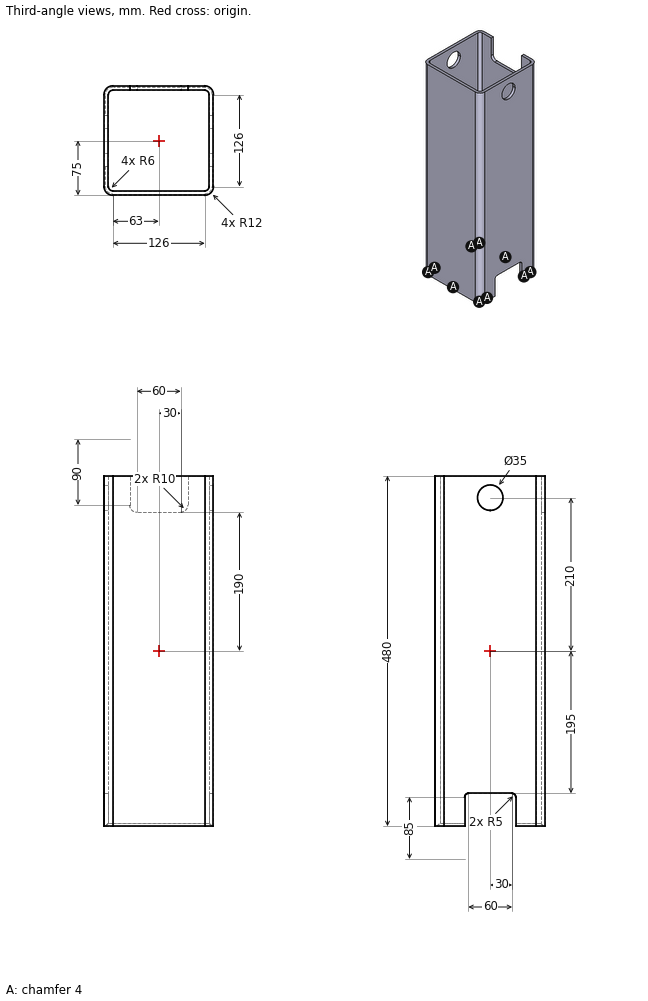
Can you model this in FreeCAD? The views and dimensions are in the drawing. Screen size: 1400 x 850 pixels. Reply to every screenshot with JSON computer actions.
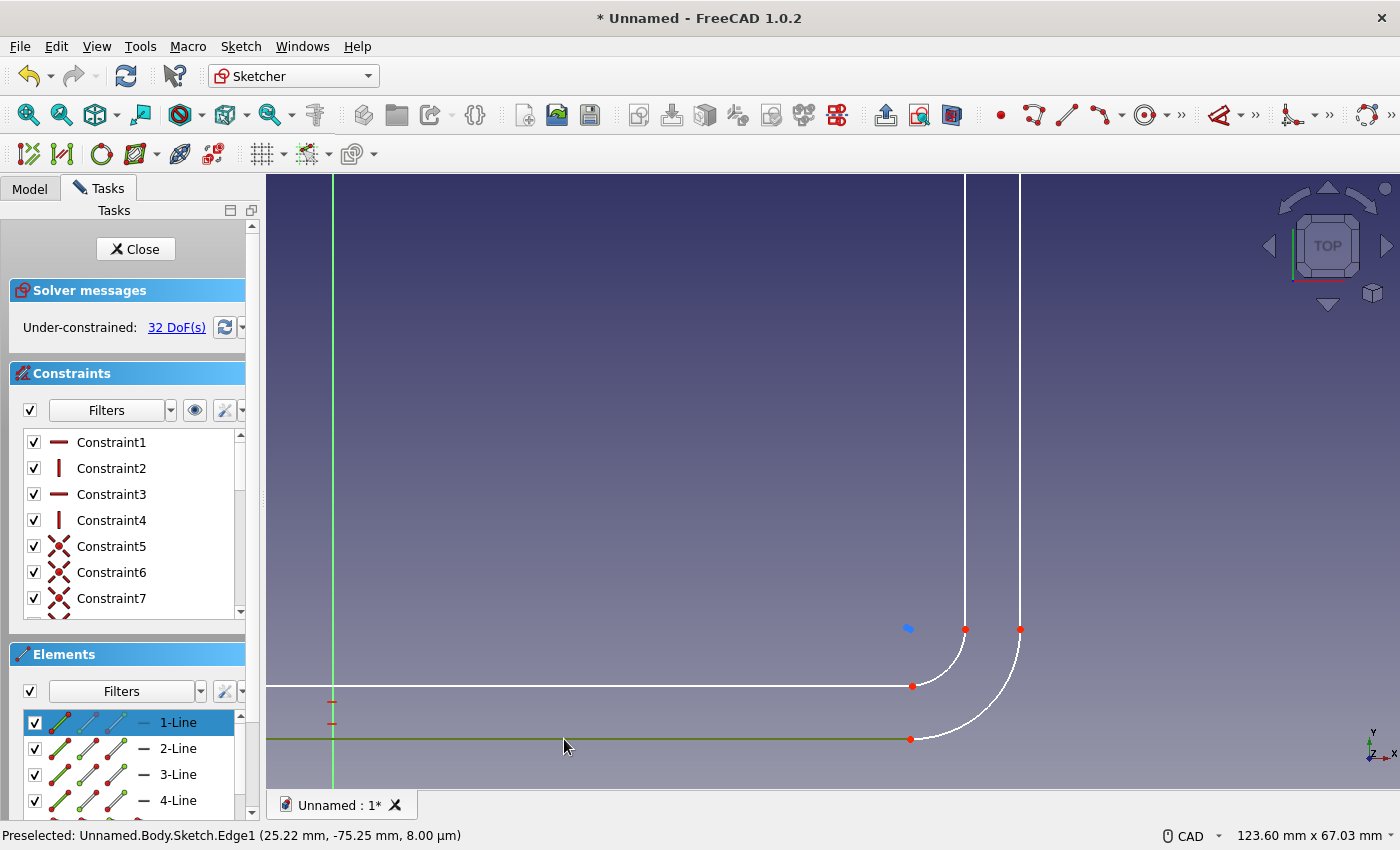
{"action": "left_click", "coordinate": [960, 727]}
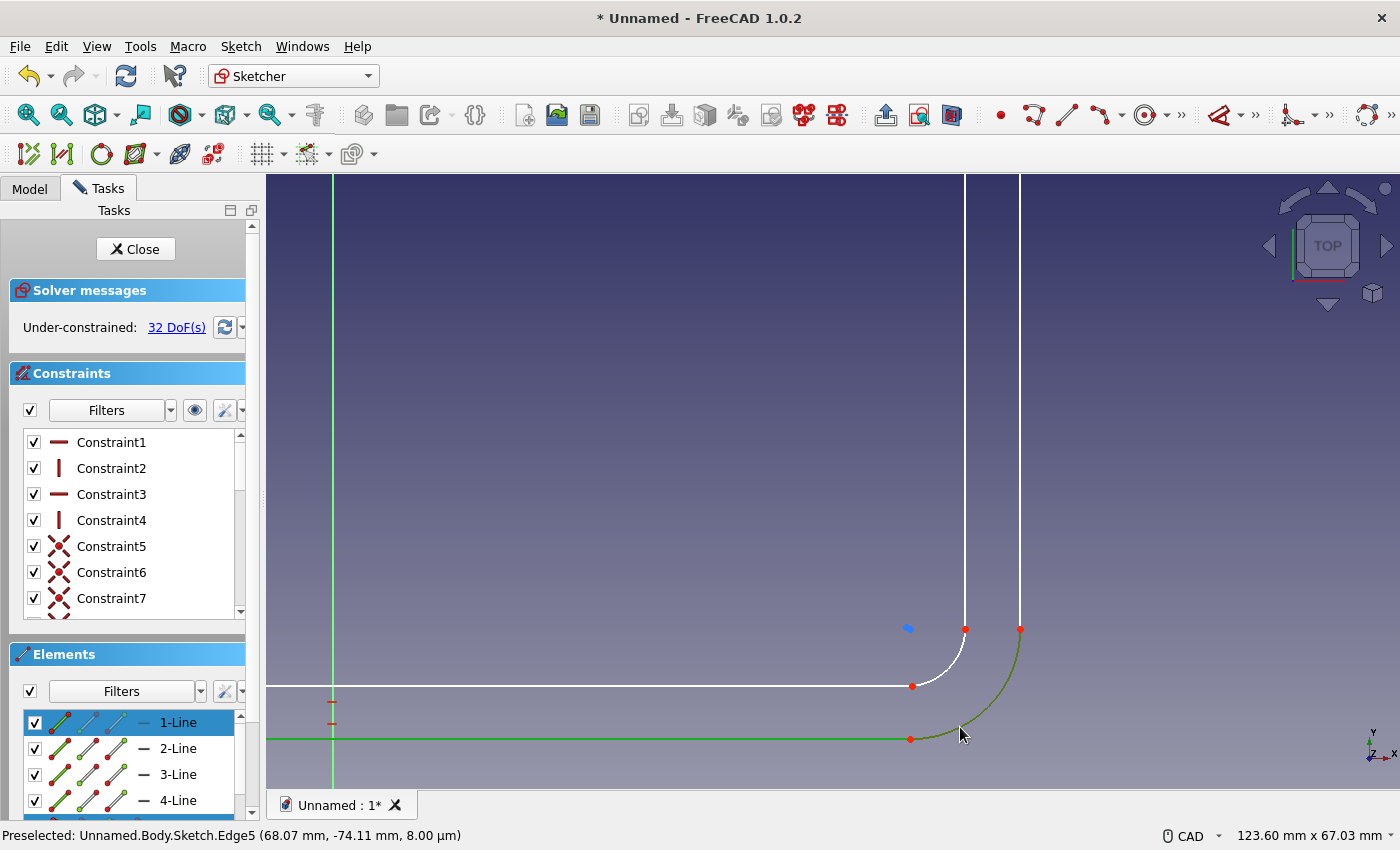
{"action": "key", "text": "t"}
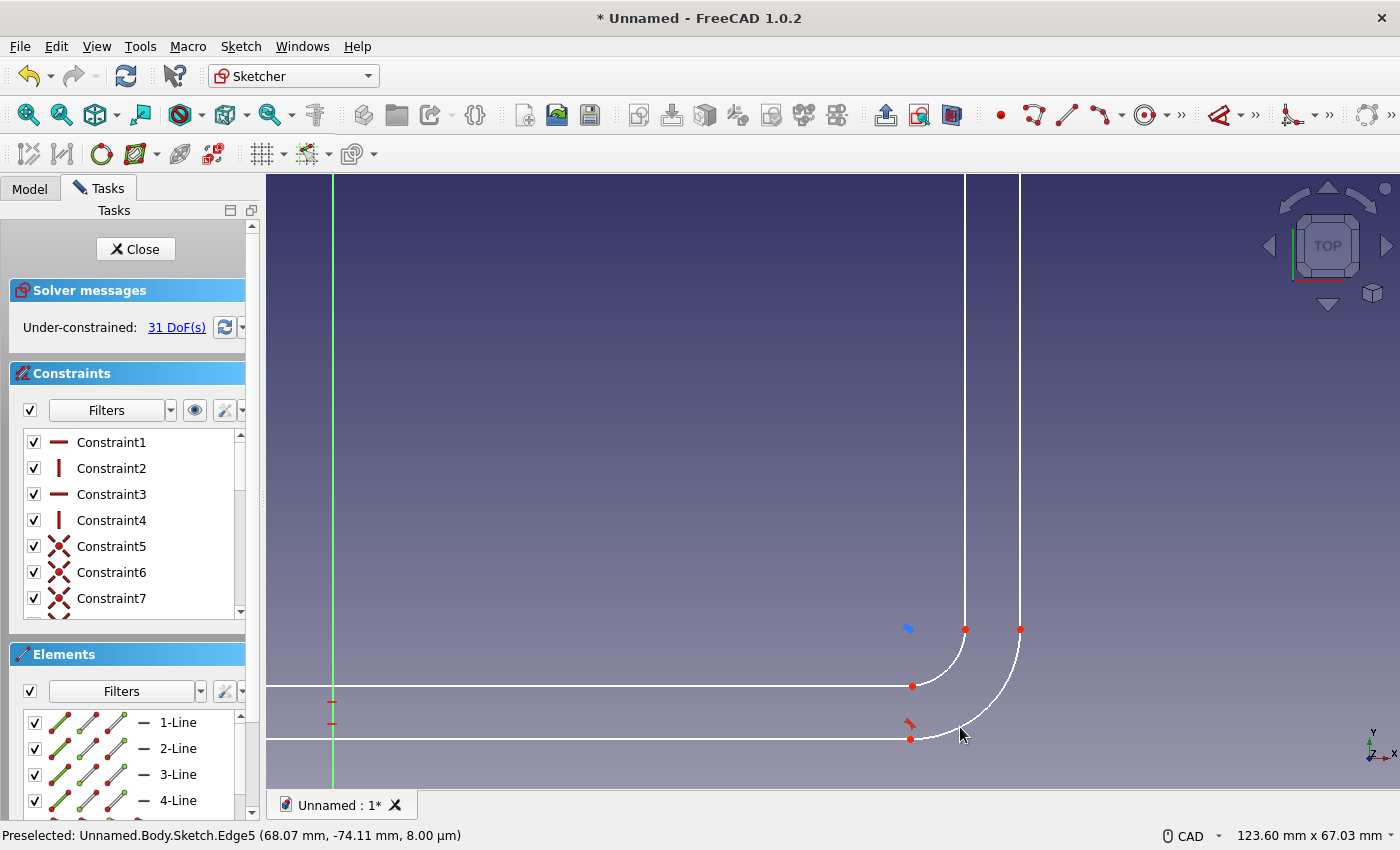
{"action": "left_click", "coordinate": [564, 739]}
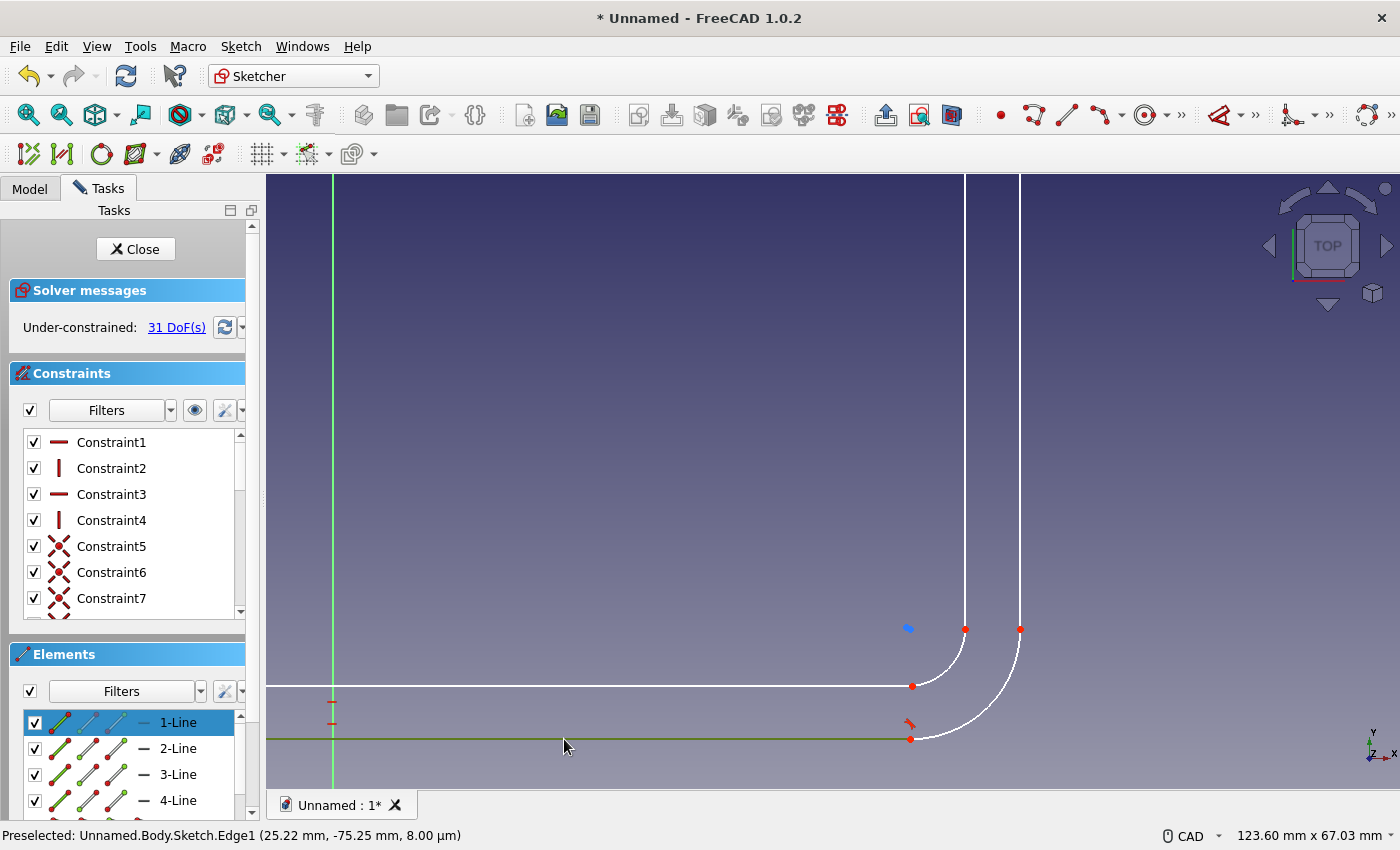
{"action": "scroll", "coordinate": [951, 668], "scroll_direction": "down", "scroll_amount": 6}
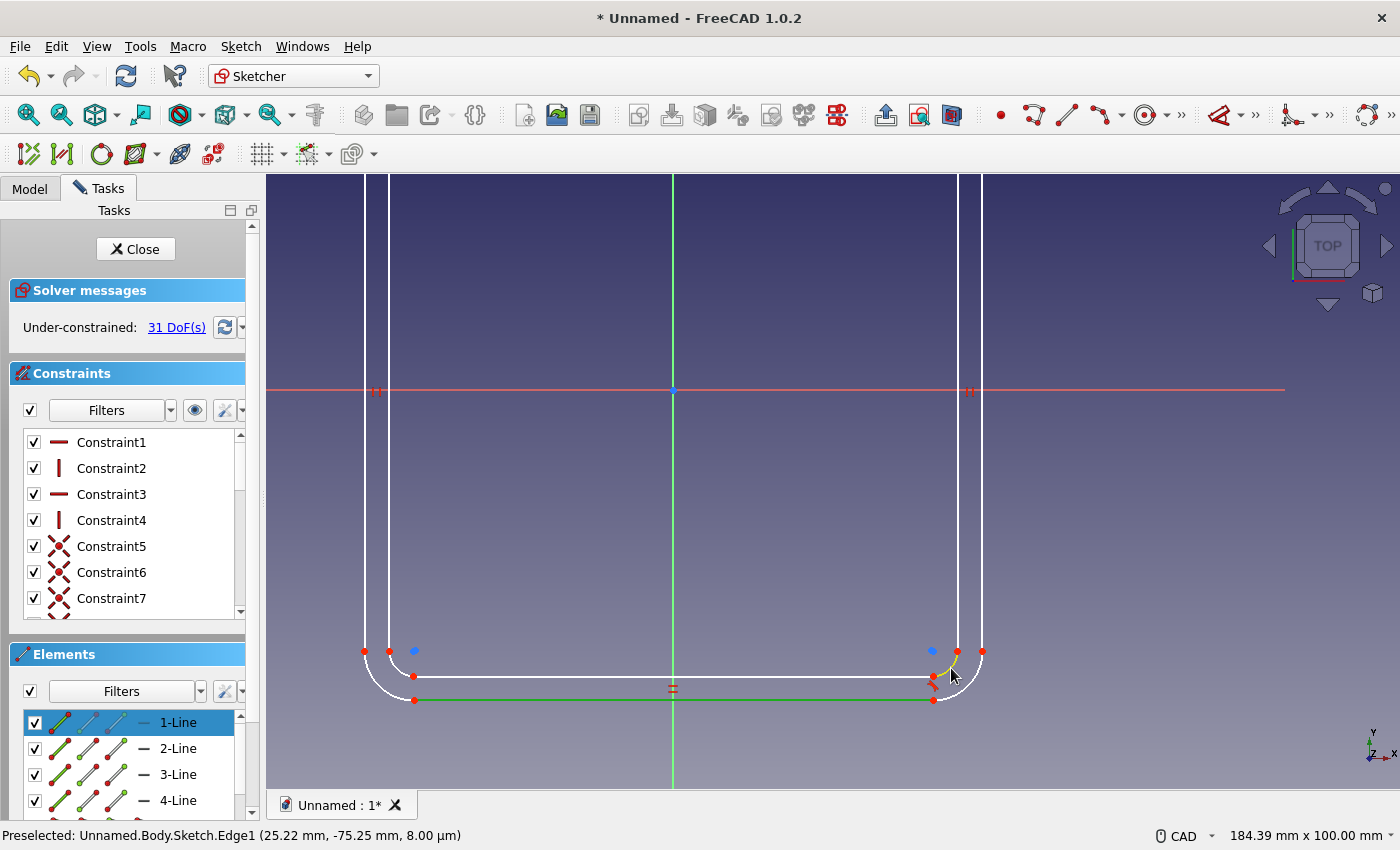
{"action": "left_click", "coordinate": [562, 672]}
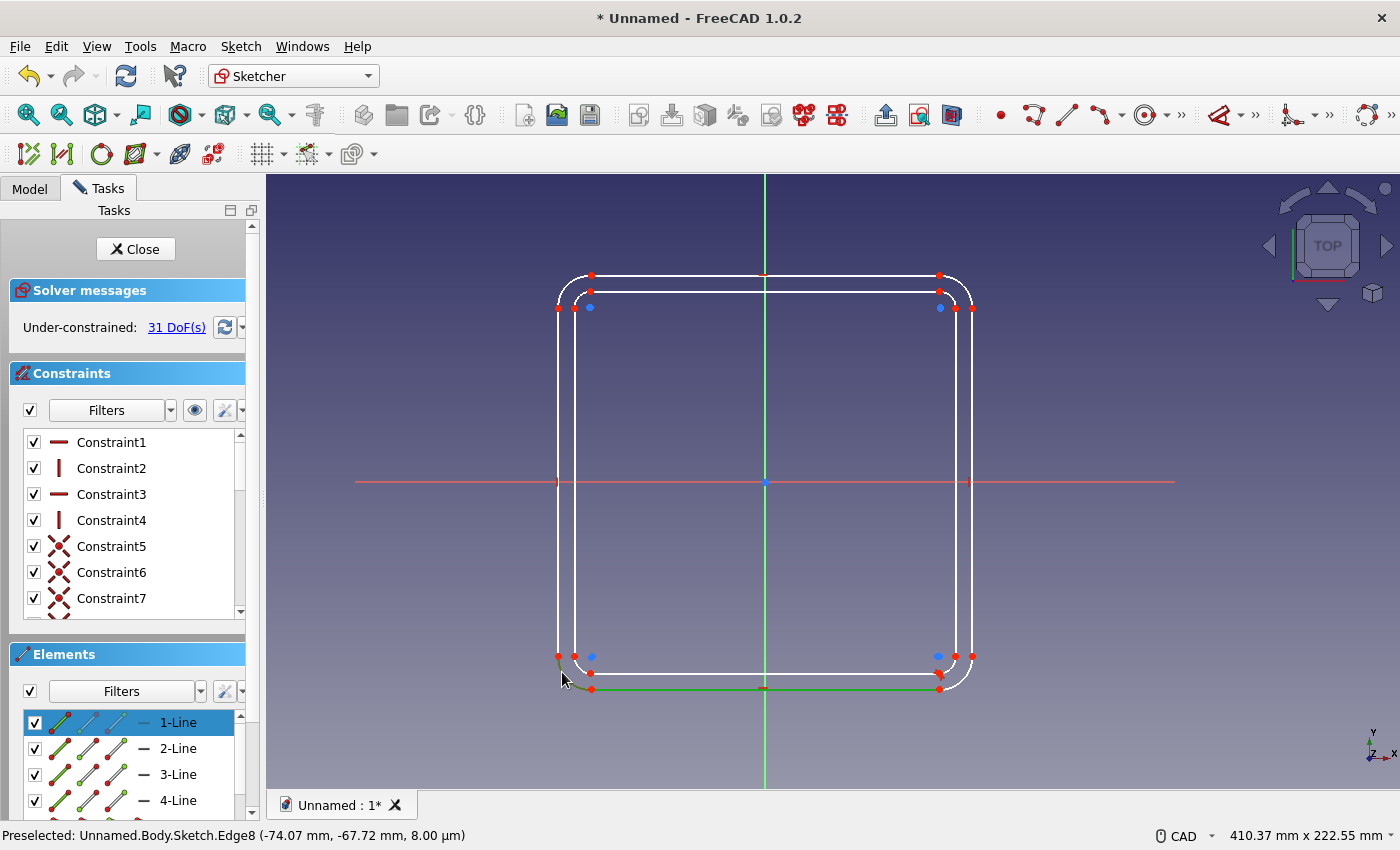
{"action": "key", "text": "t"}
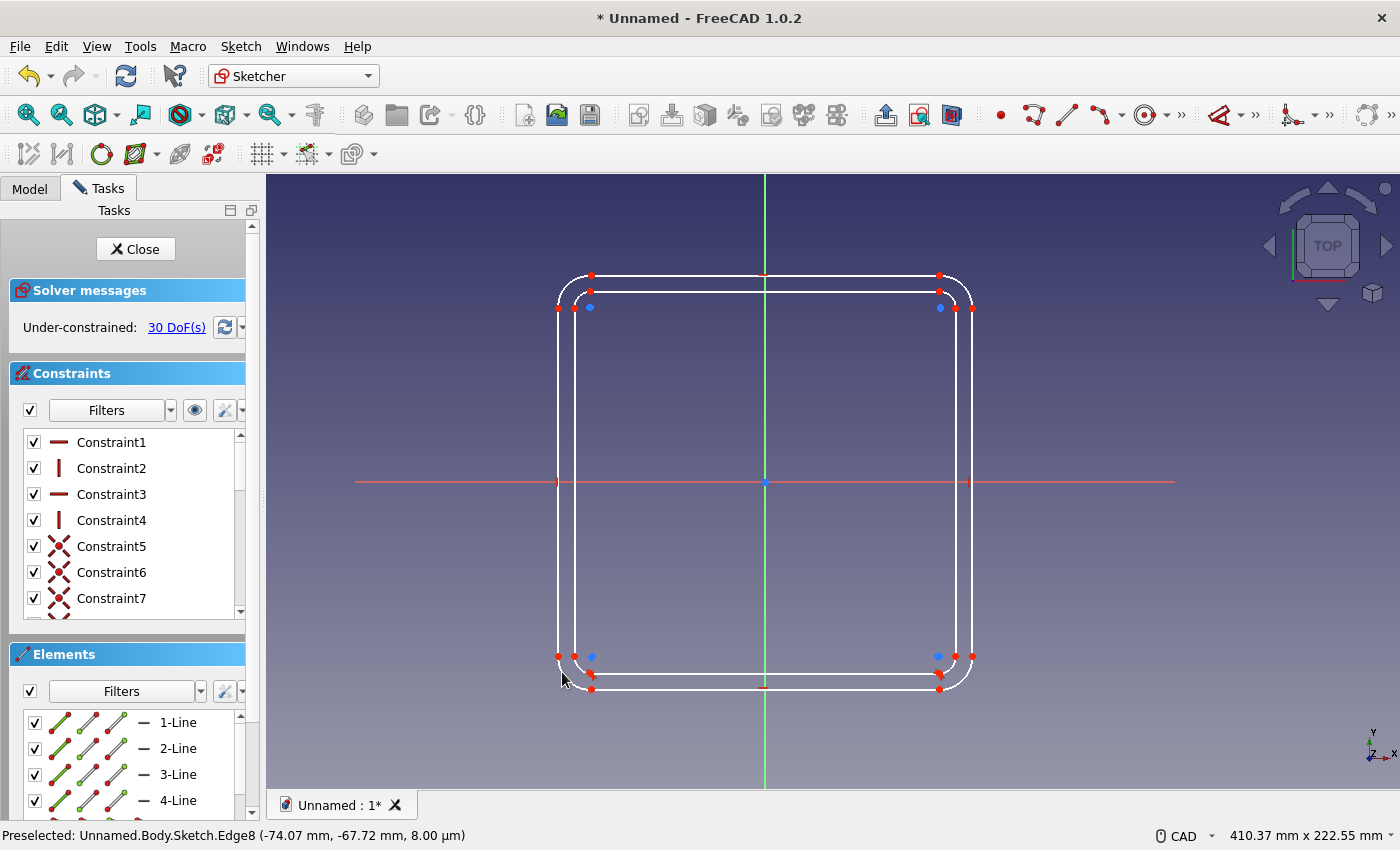
{"action": "left_click", "coordinate": [972, 553]}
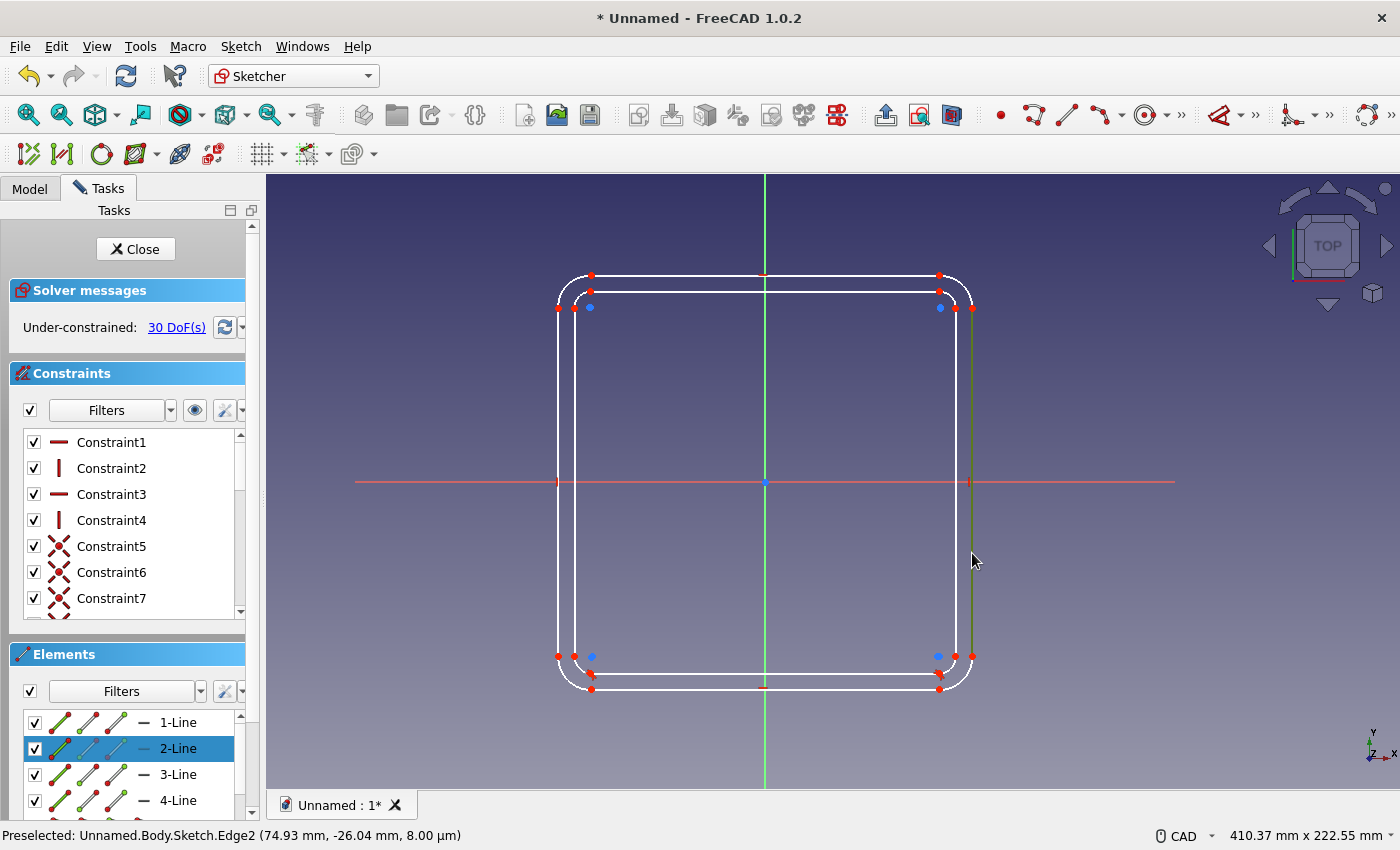
{"action": "left_click", "coordinate": [954, 686]}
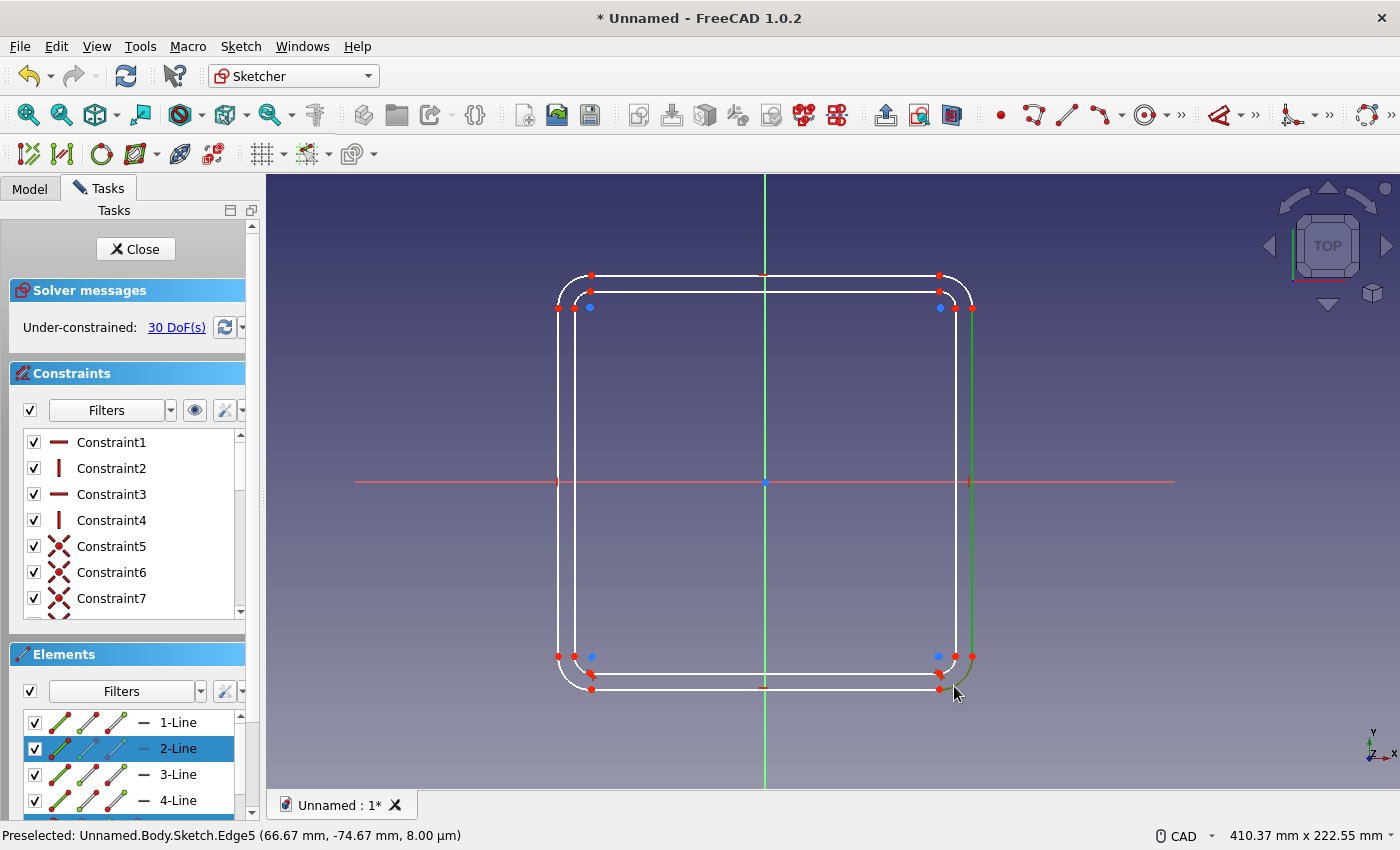
{"action": "key", "text": "t"}